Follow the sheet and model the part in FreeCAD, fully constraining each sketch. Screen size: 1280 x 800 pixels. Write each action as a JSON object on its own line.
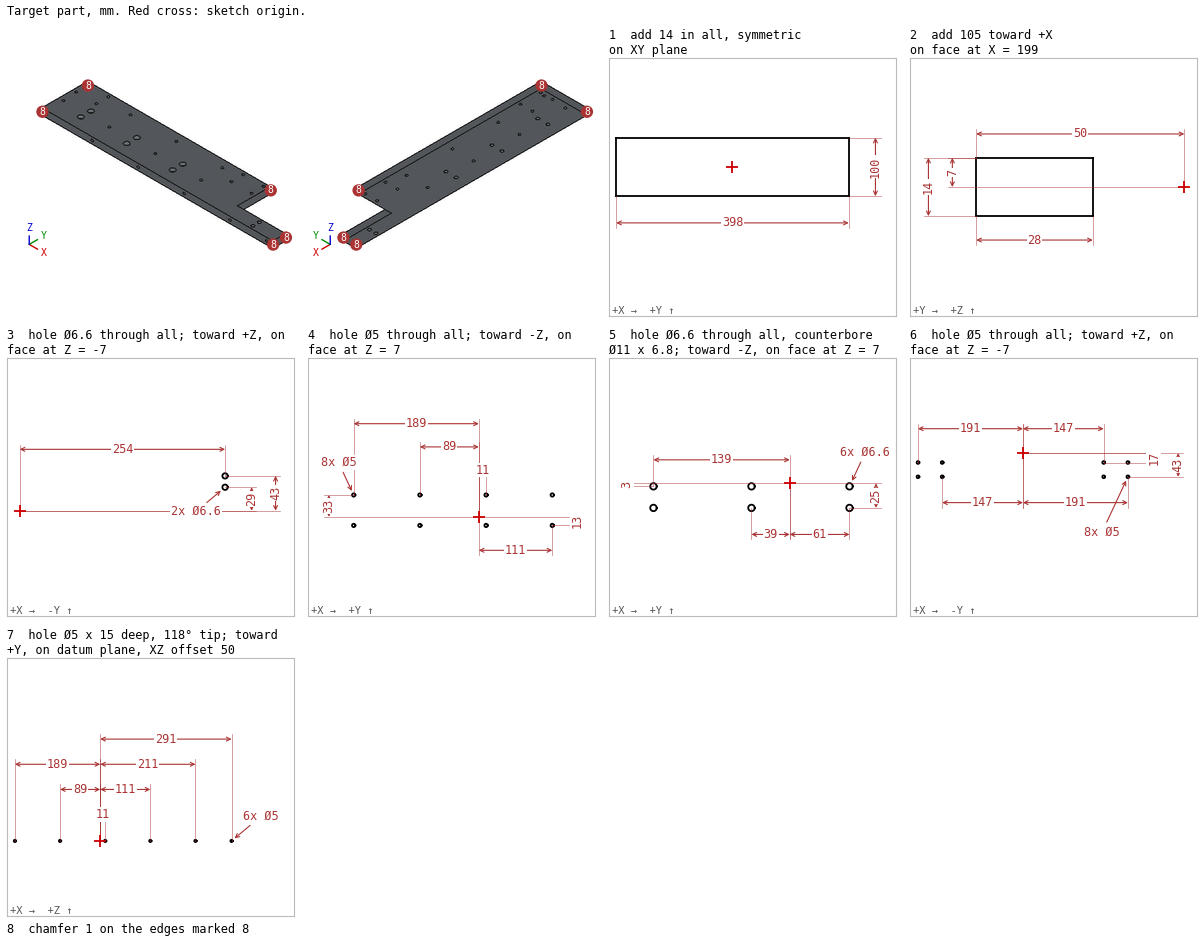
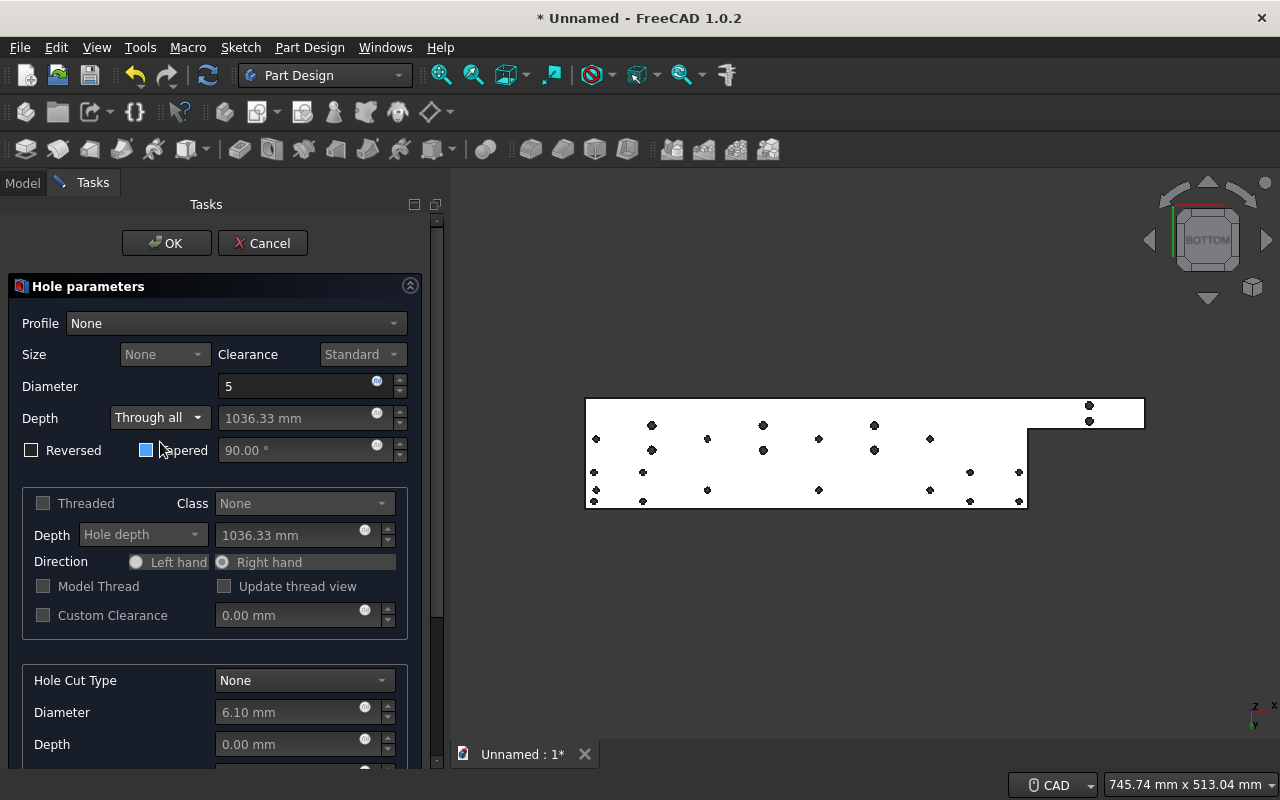
{"action": "left_click", "coordinate": [167, 243]}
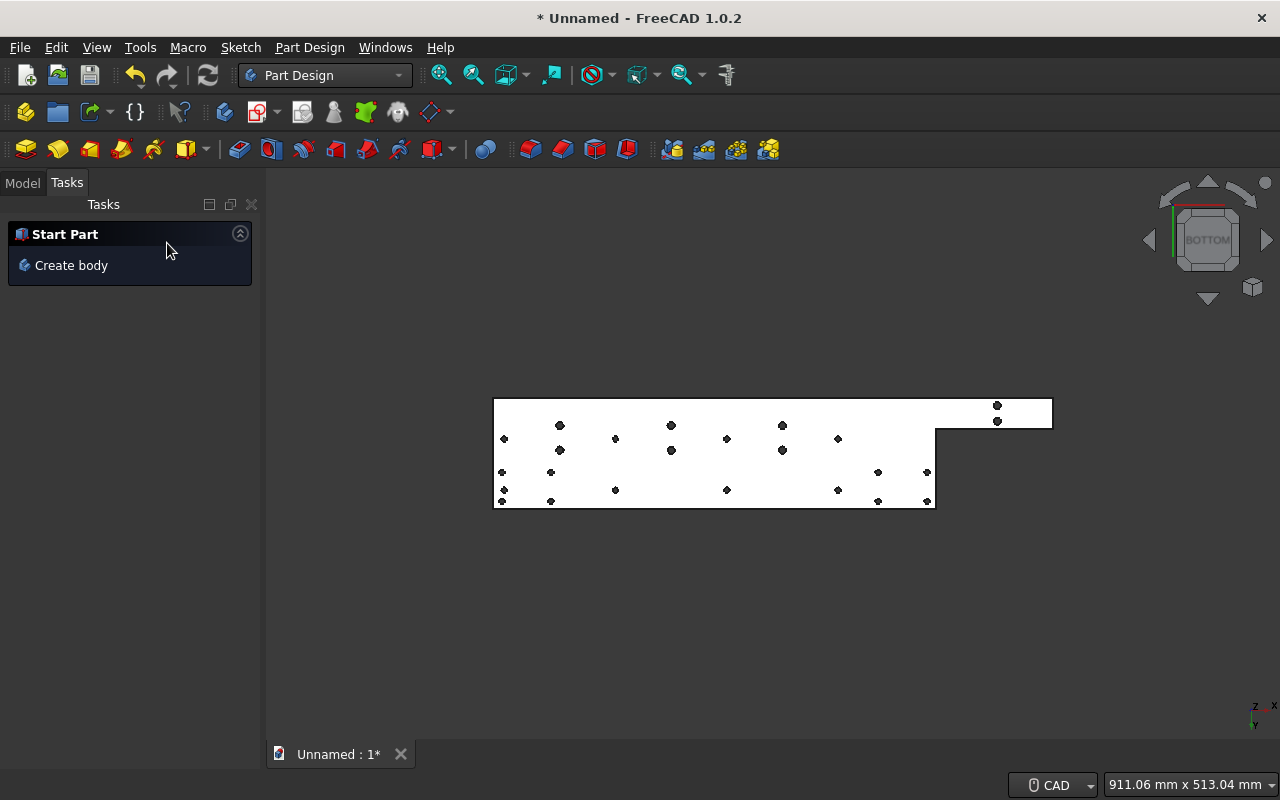
{"action": "key", "text": "0"}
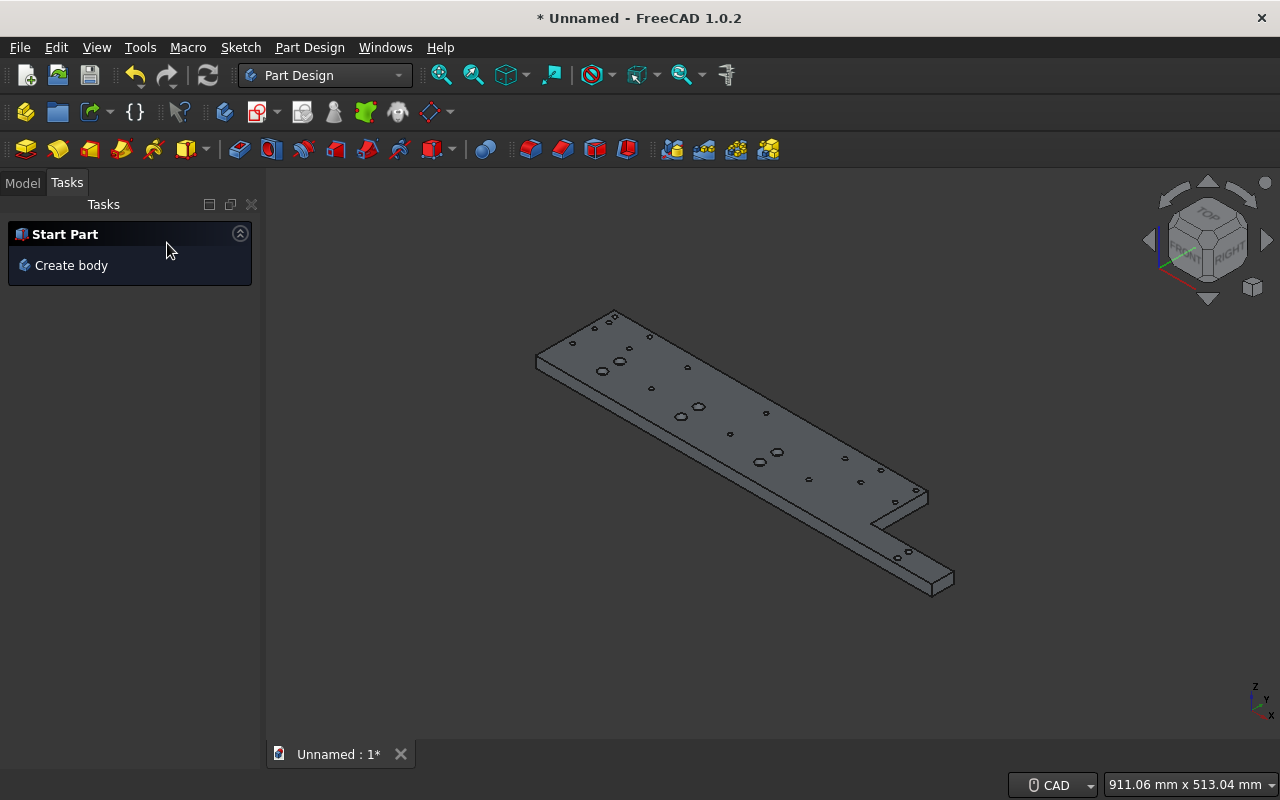
{"action": "key", "text": "1"}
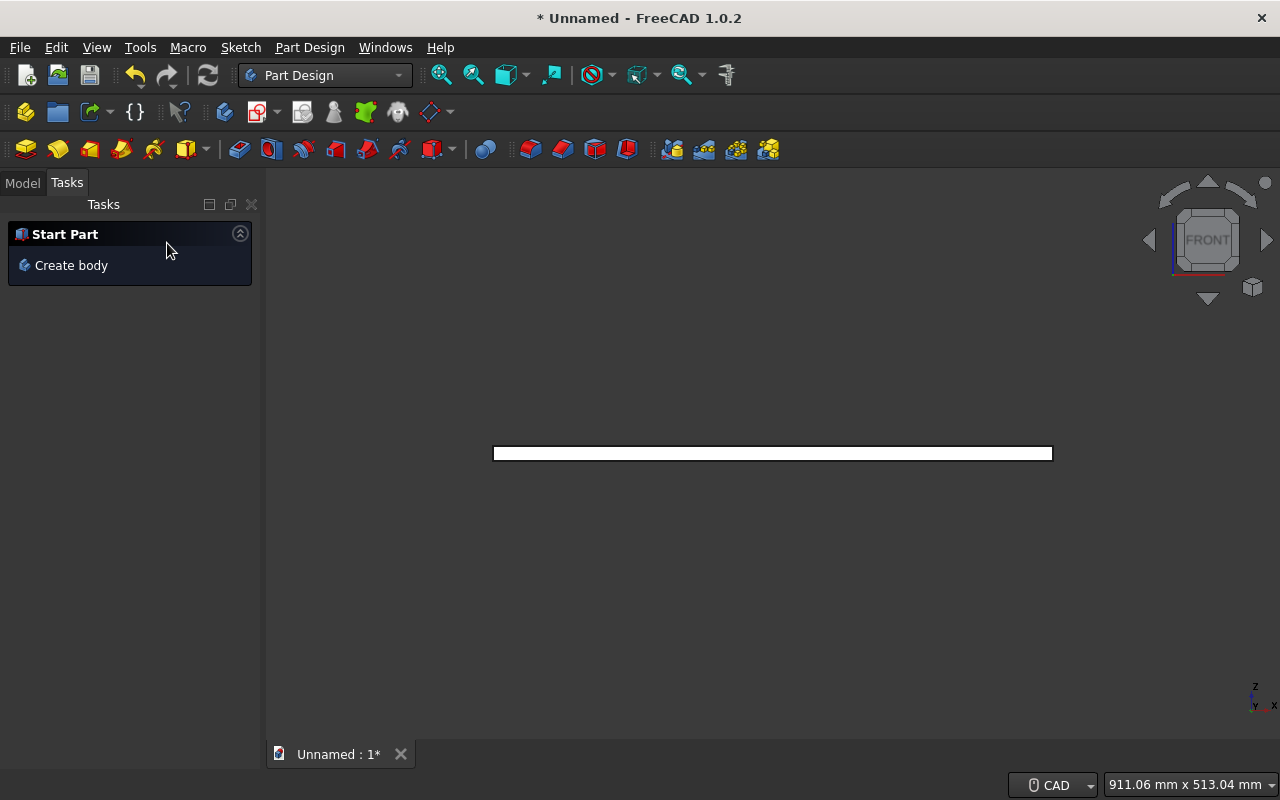
{"action": "key", "text": "2"}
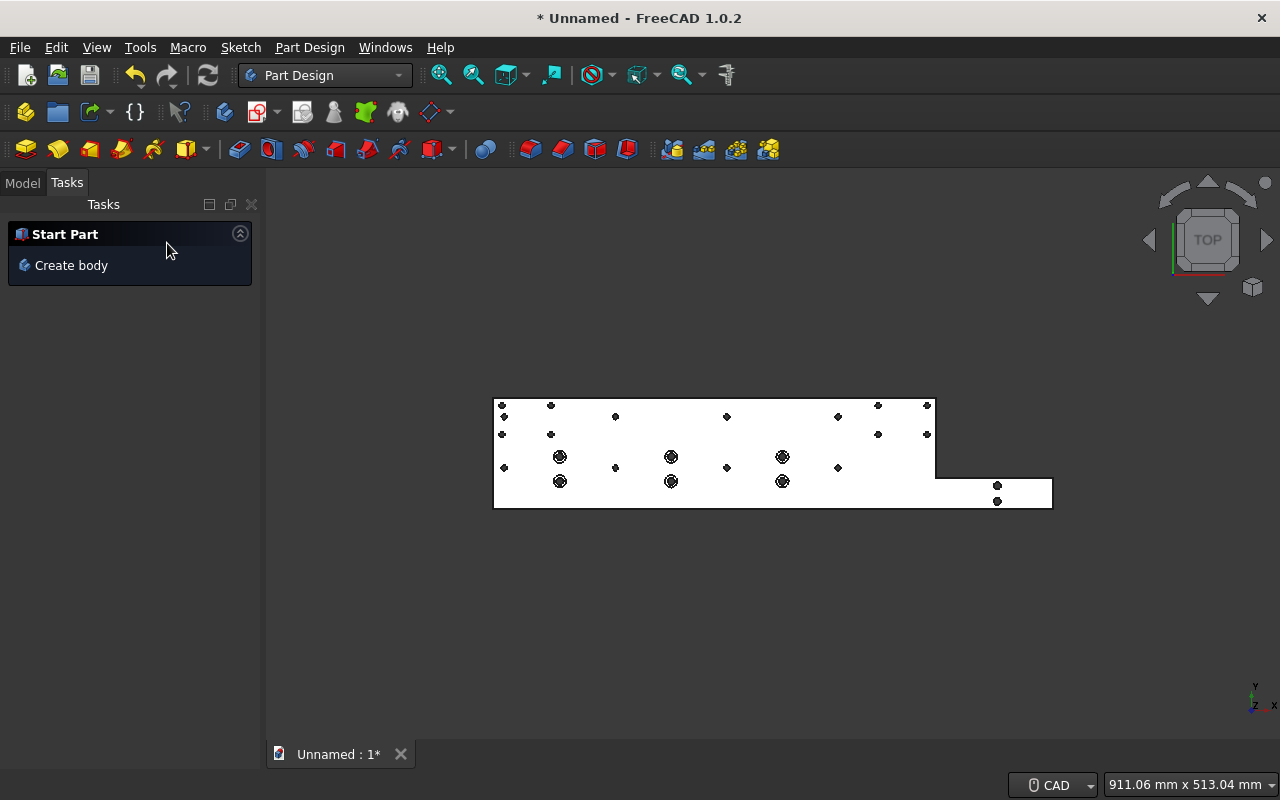
{"action": "left_click", "coordinate": [23, 182]}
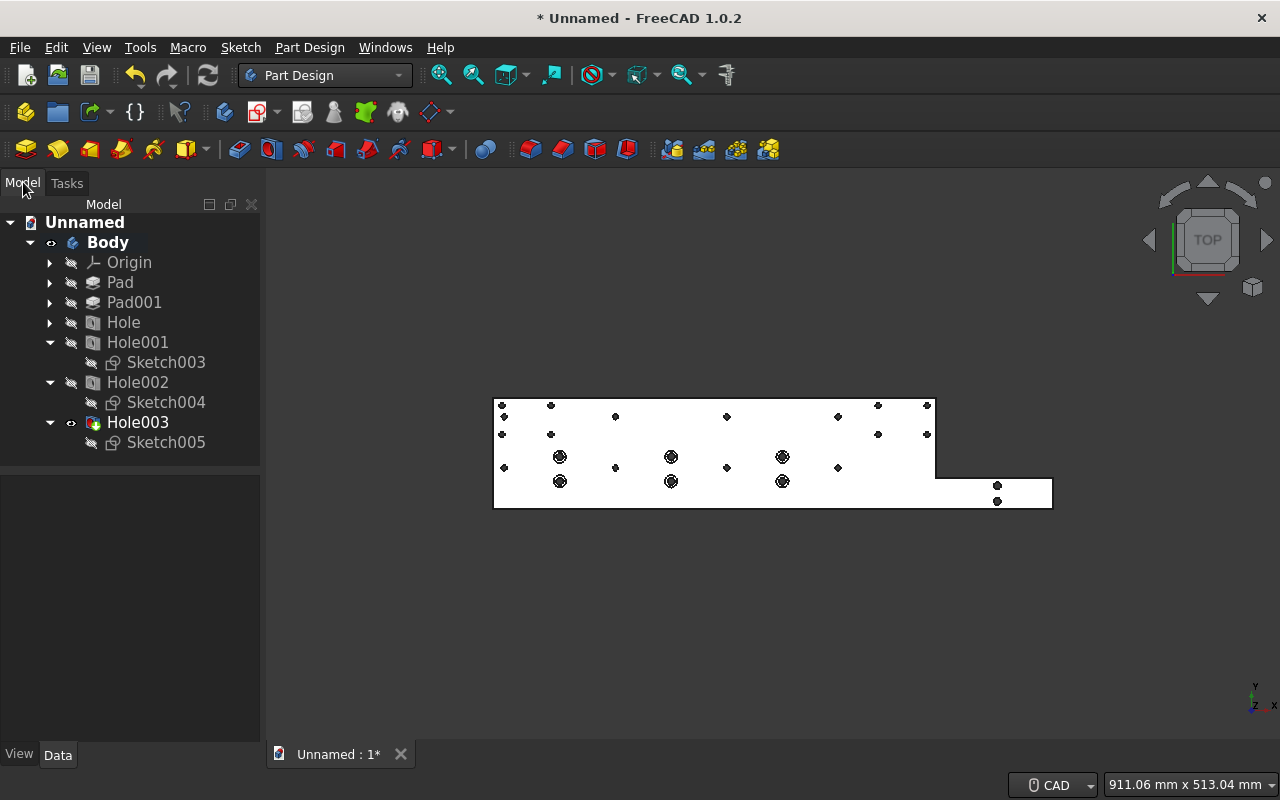
{"action": "left_click", "coordinate": [50, 263]}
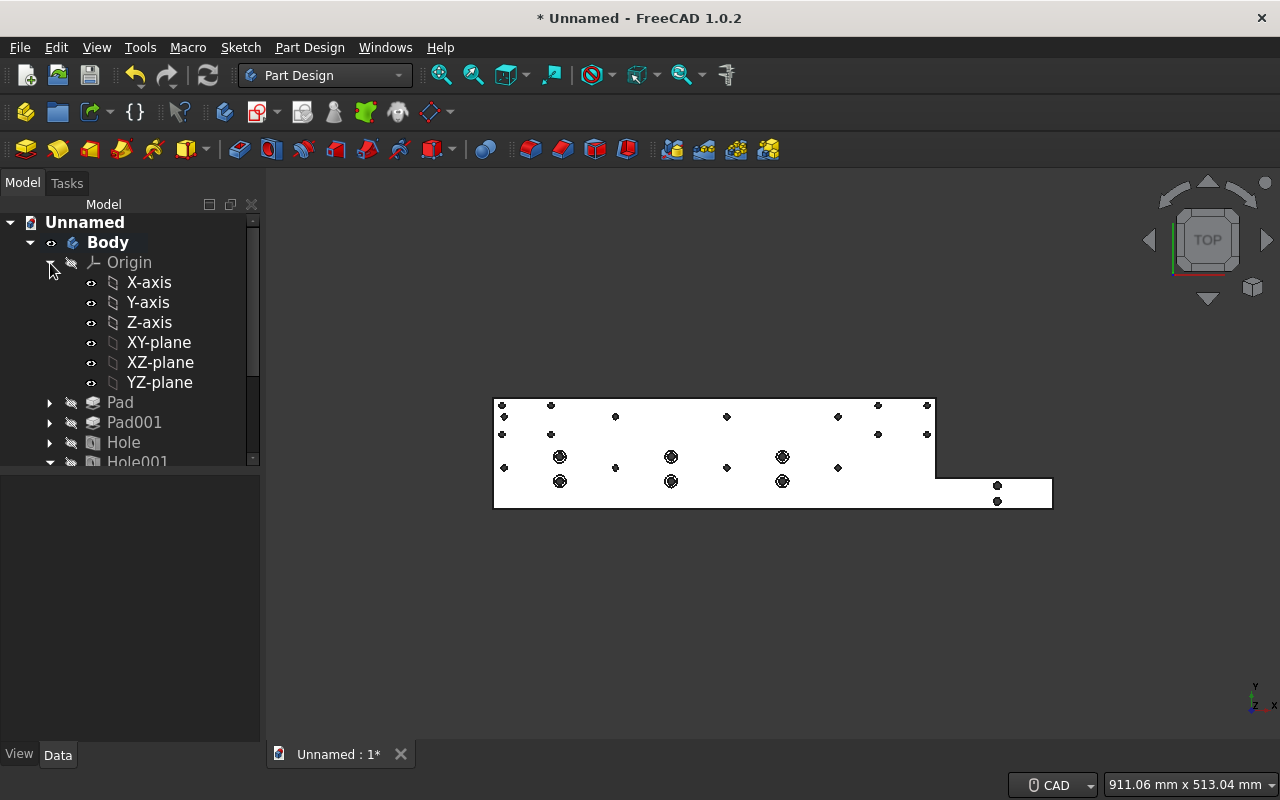
{"action": "left_click", "coordinate": [136, 363]}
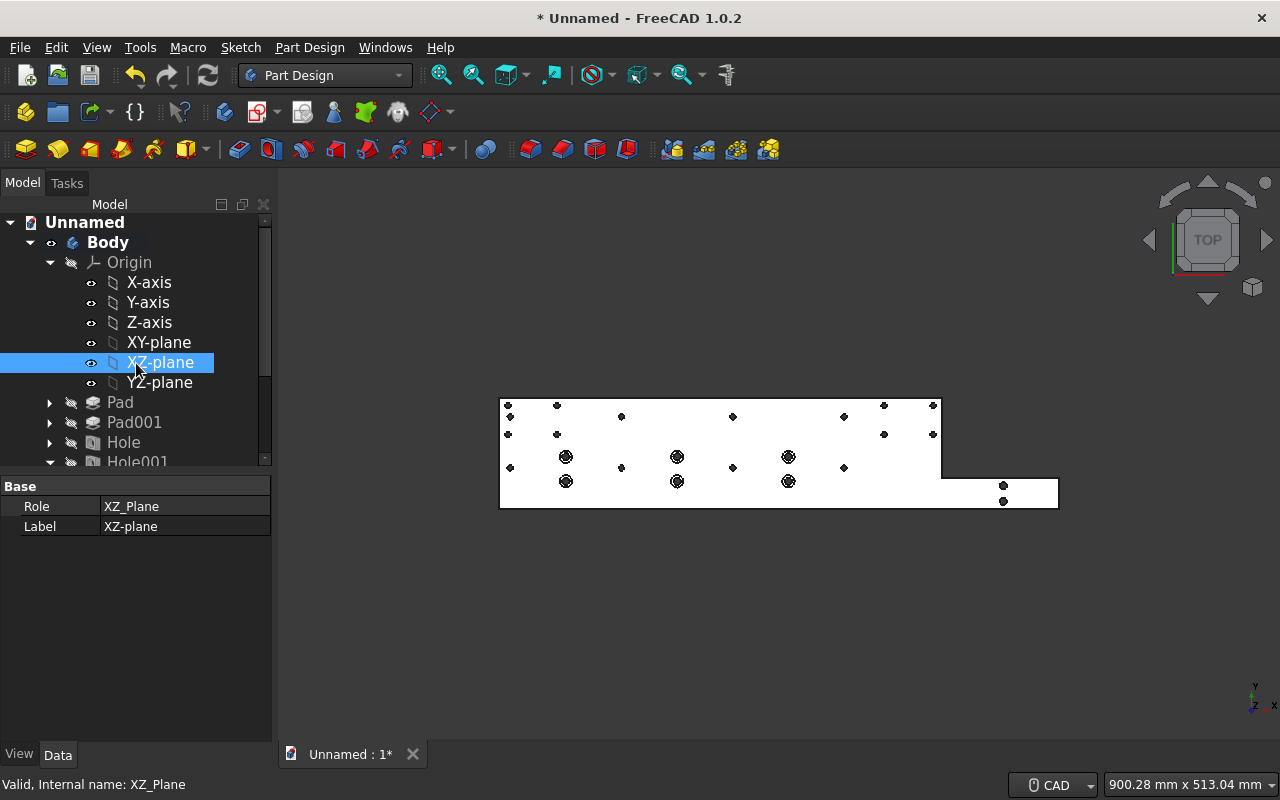
{"action": "left_click", "coordinate": [430, 112]}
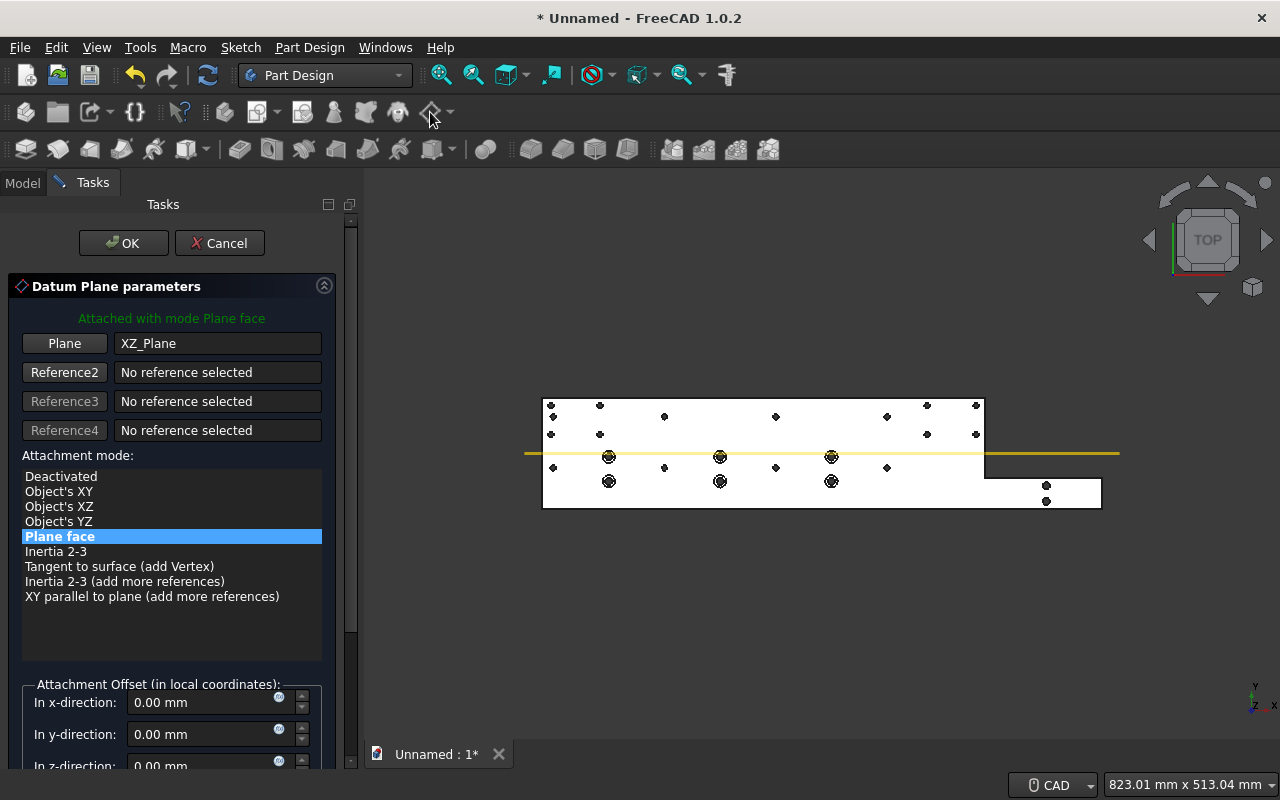
{"action": "scroll", "coordinate": [351, 491], "scroll_direction": "down", "scroll_amount": 2}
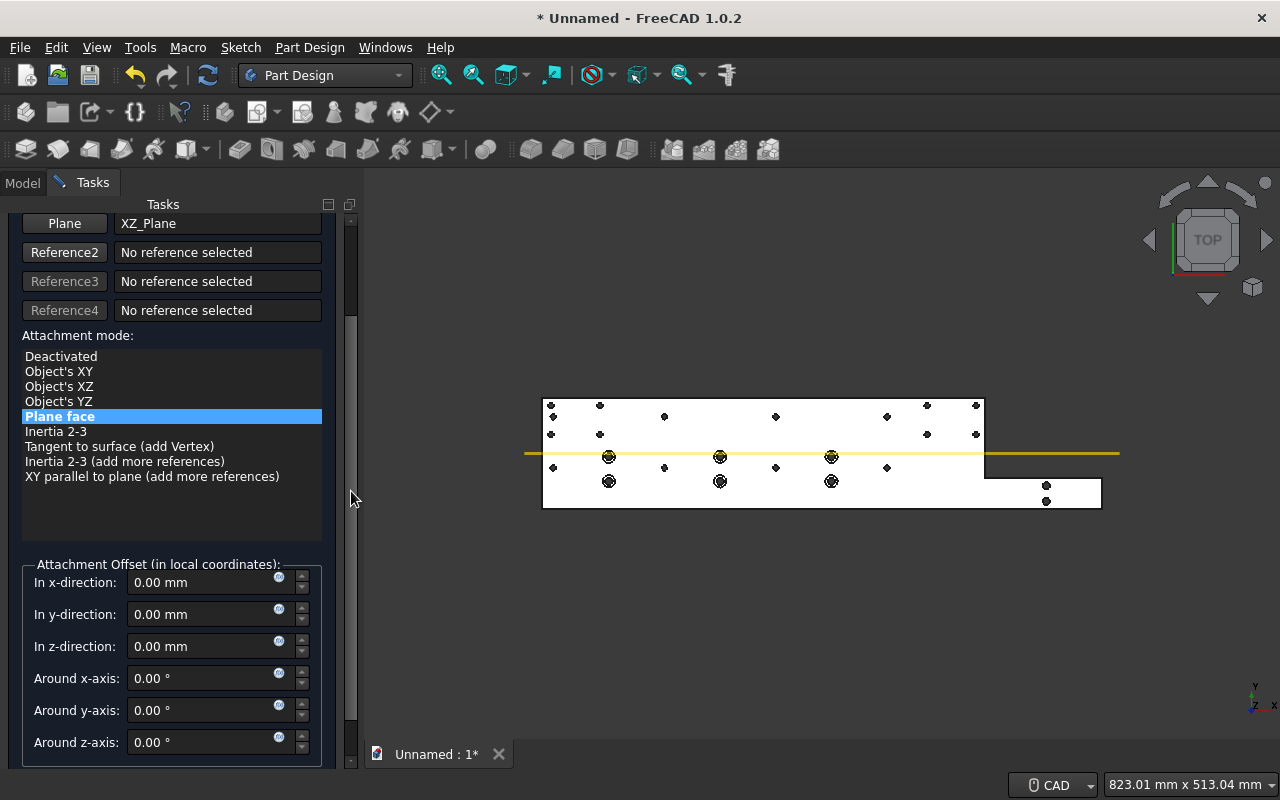
{"action": "triple_click", "coordinate": [210, 646]}